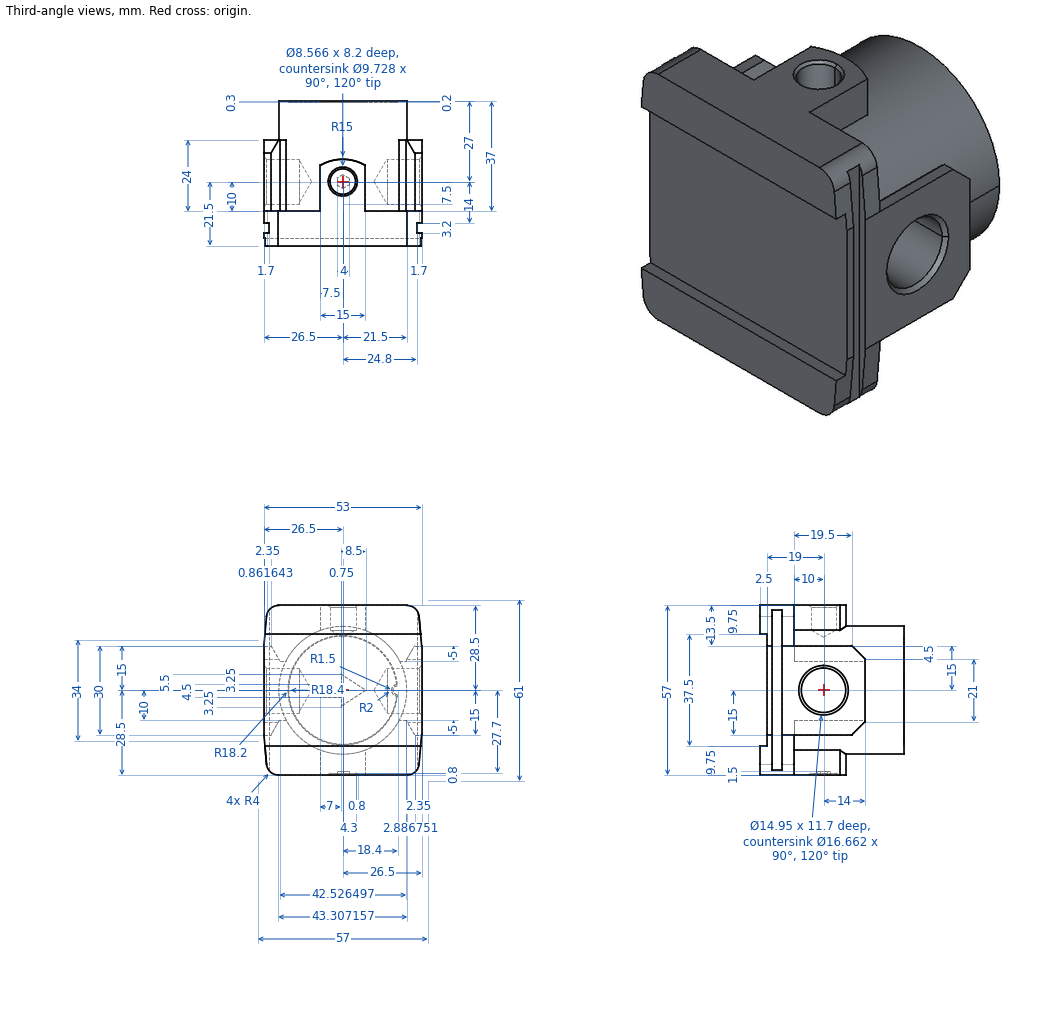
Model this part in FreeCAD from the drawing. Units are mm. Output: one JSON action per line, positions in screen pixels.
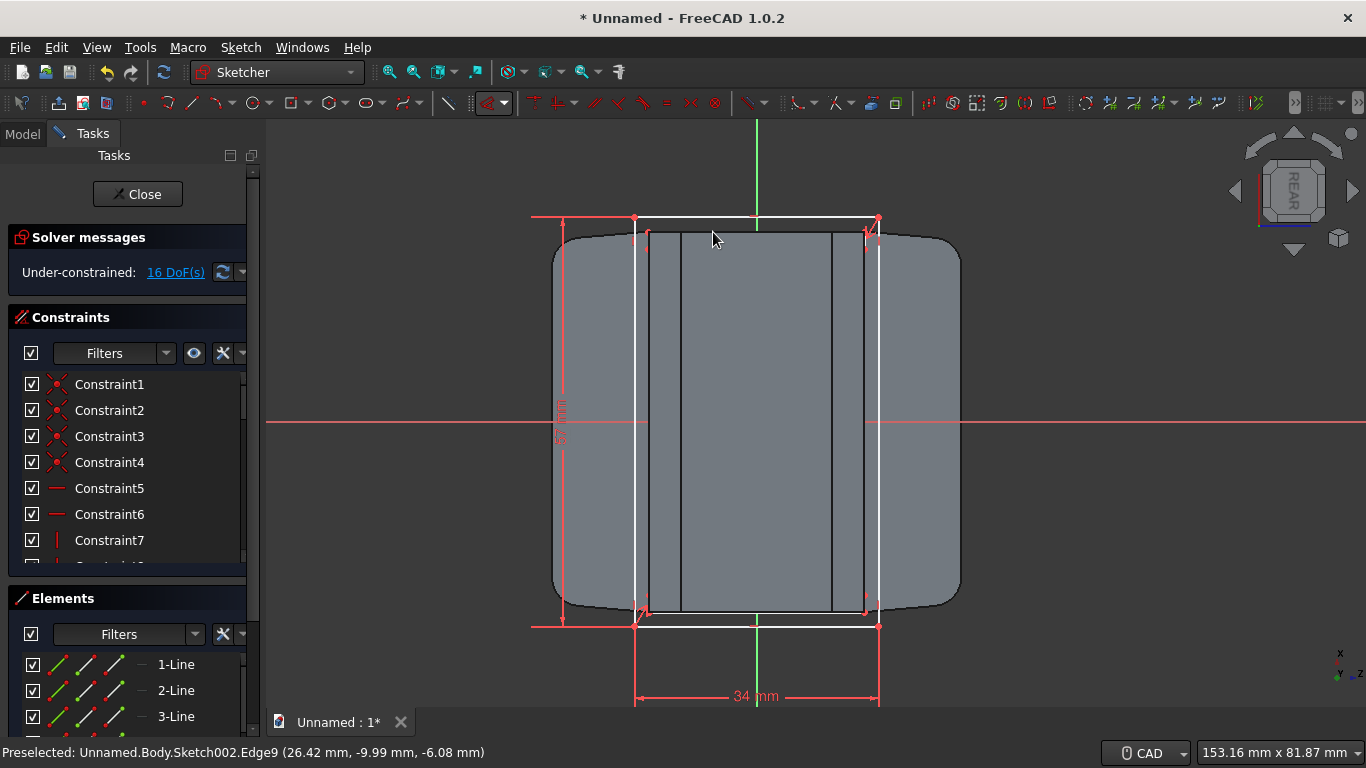
{"action": "left_click", "coordinate": [506, 104]}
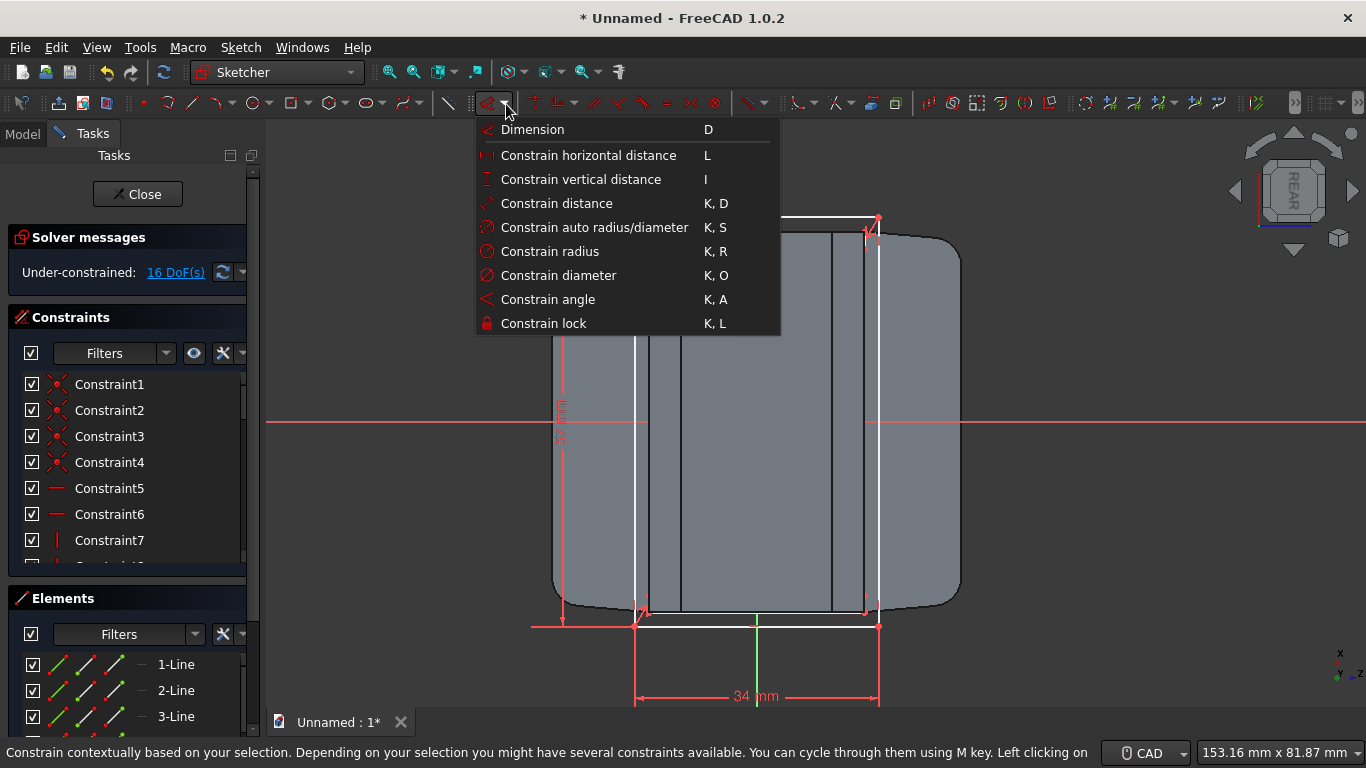
{"action": "left_click", "coordinate": [628, 155]}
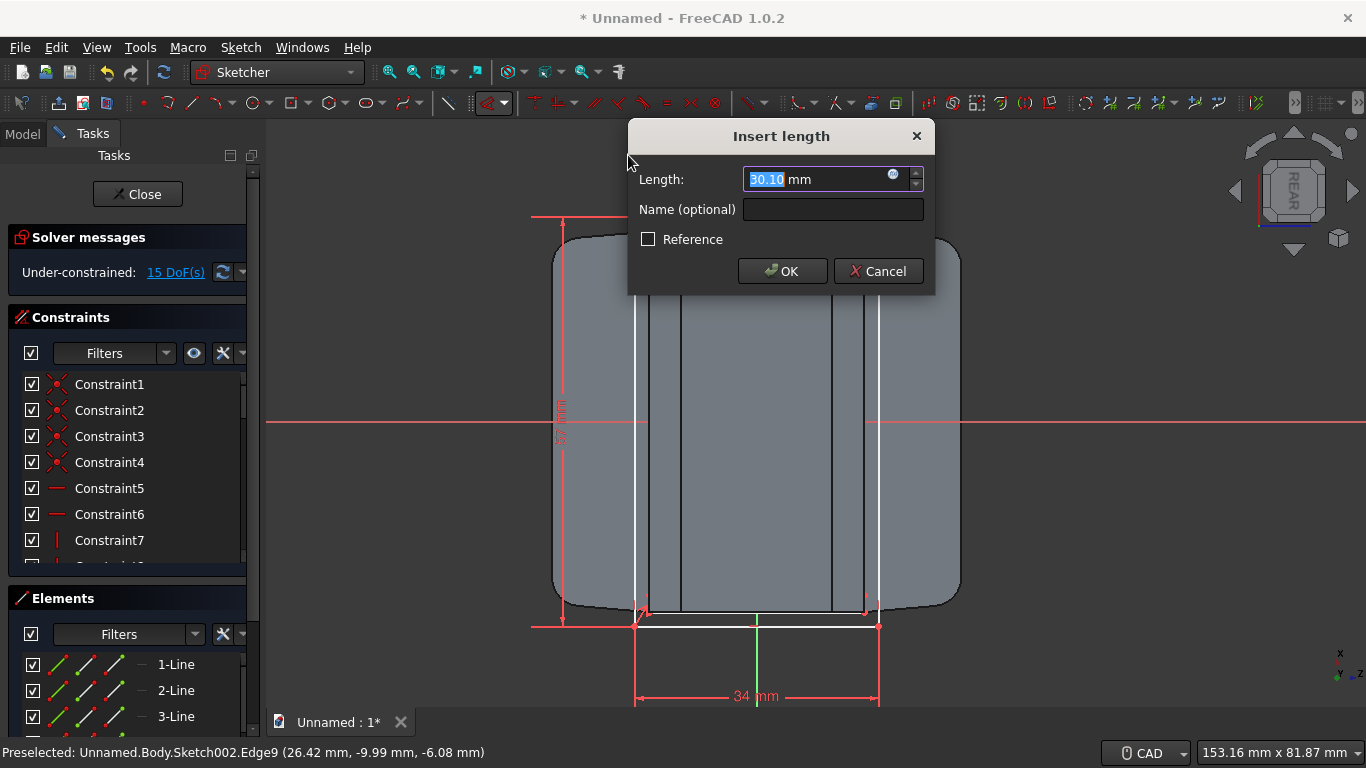
{"action": "type", "text": "30"}
{"action": "key", "text": "Return"}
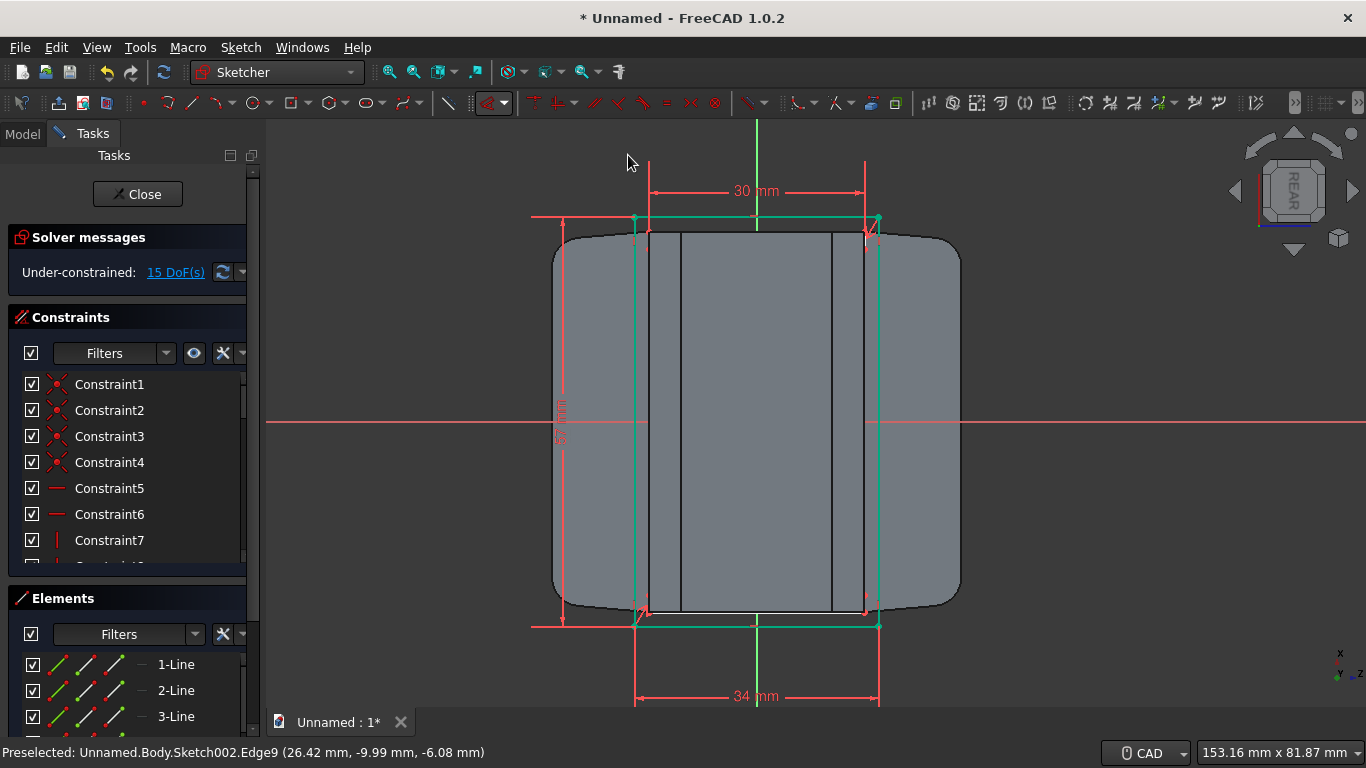
{"action": "left_click", "coordinate": [800, 613]}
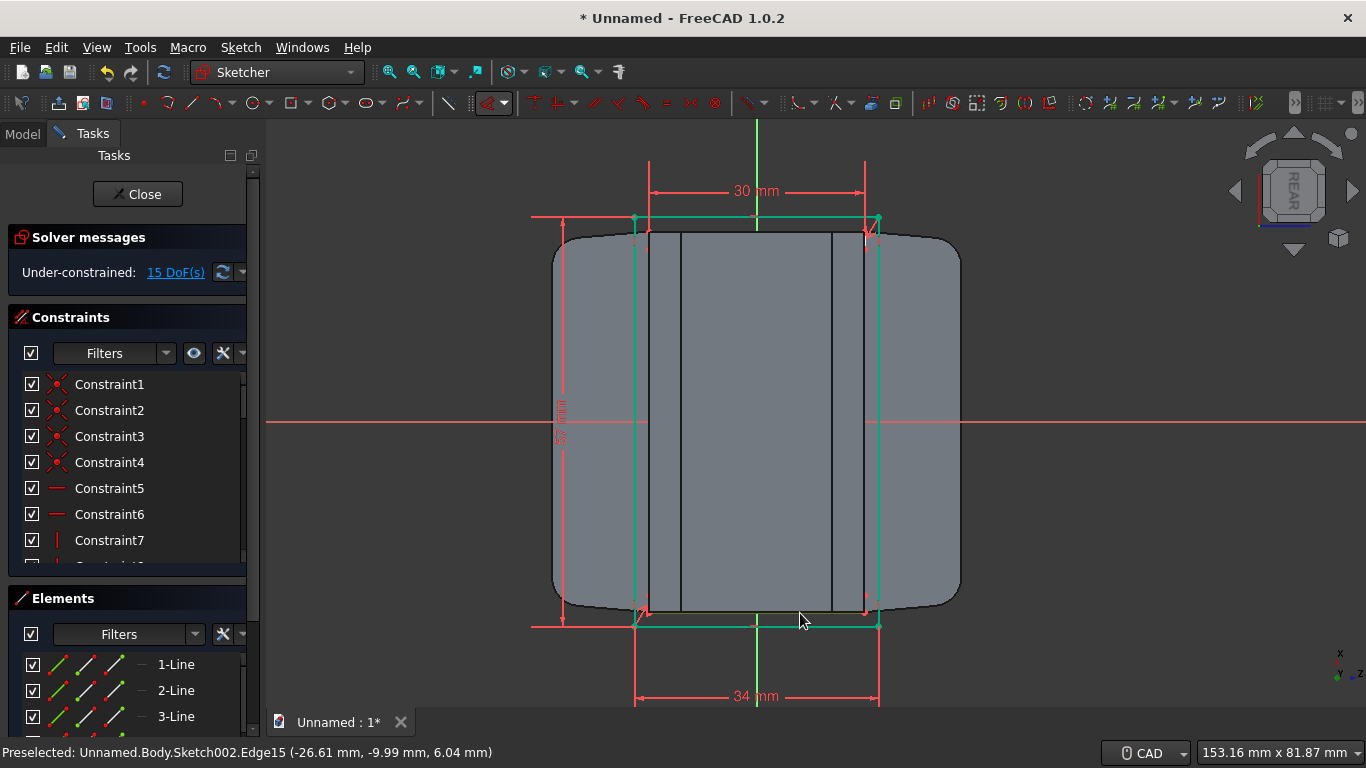
{"action": "left_click", "coordinate": [506, 104]}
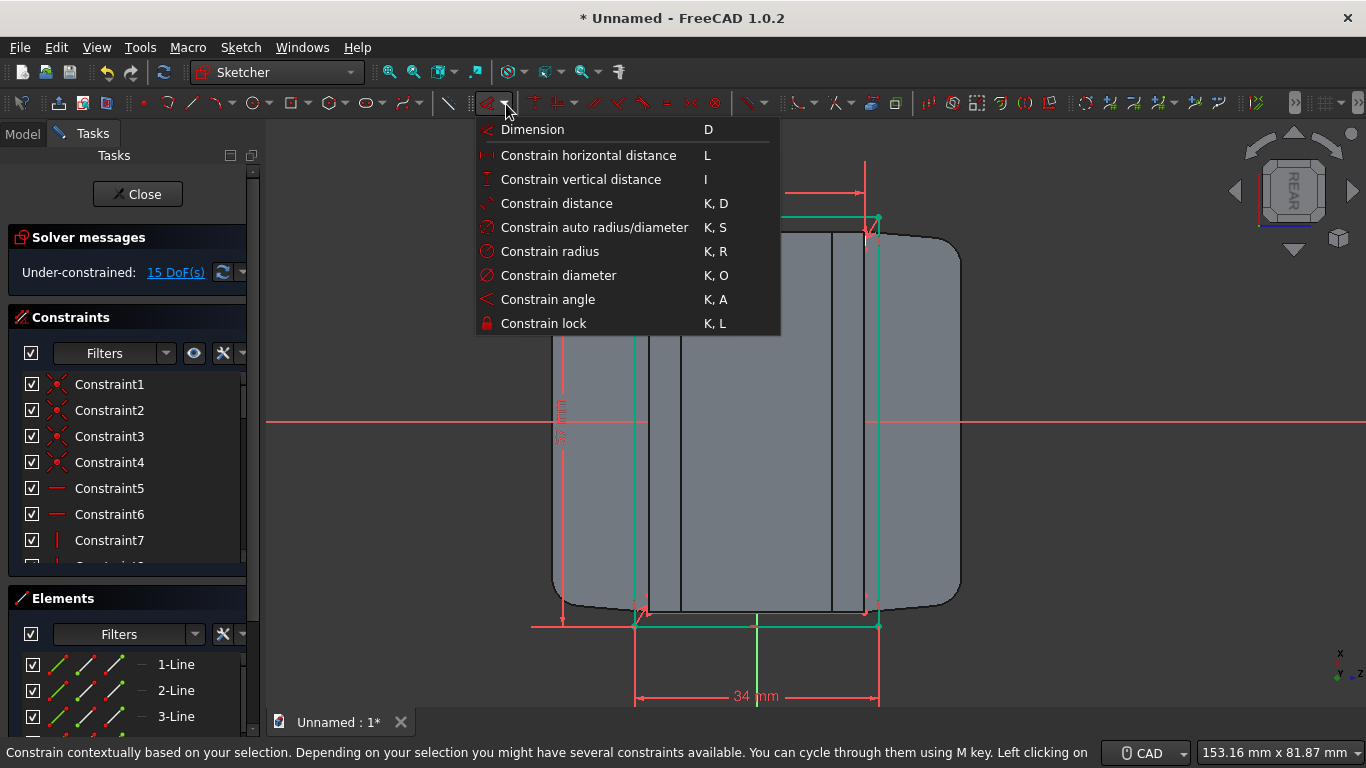
{"action": "left_click", "coordinate": [628, 155]}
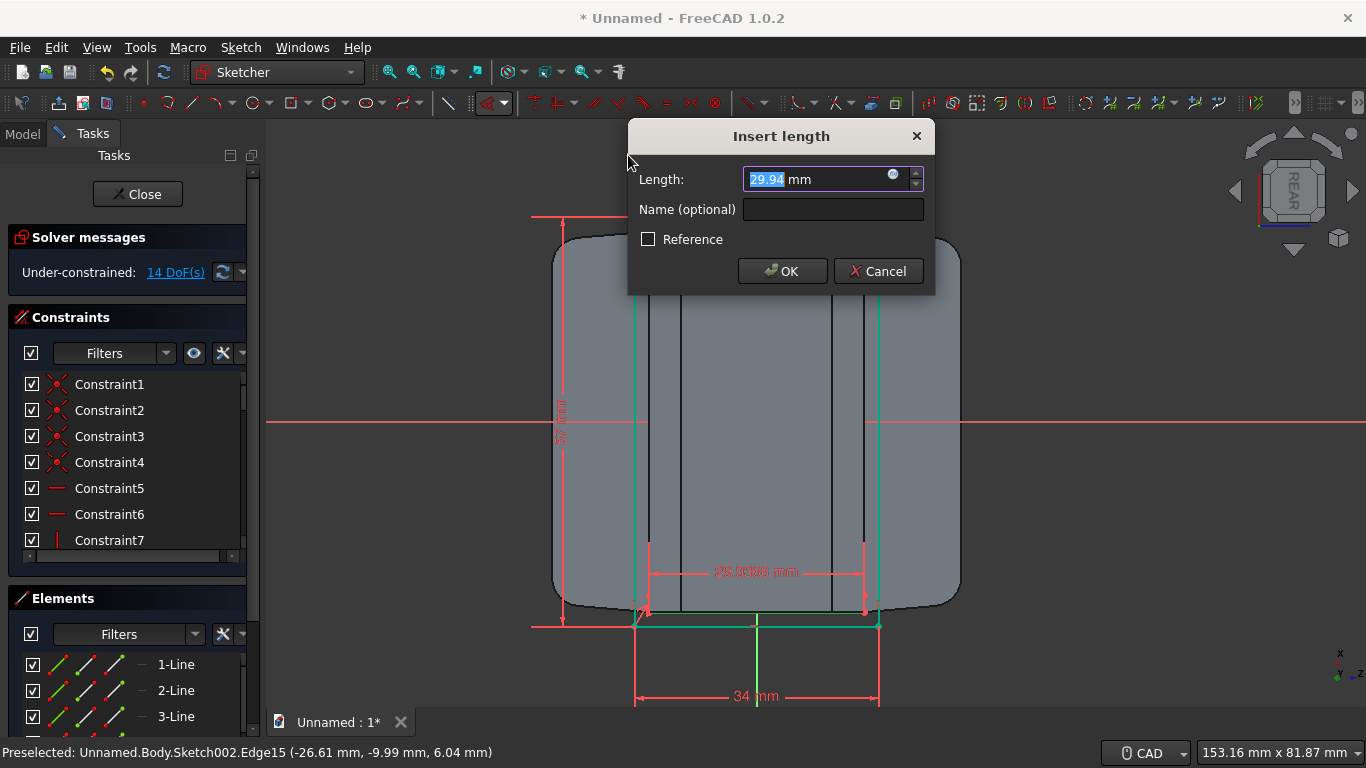
{"action": "type", "text": "30"}
{"action": "key", "text": "Return"}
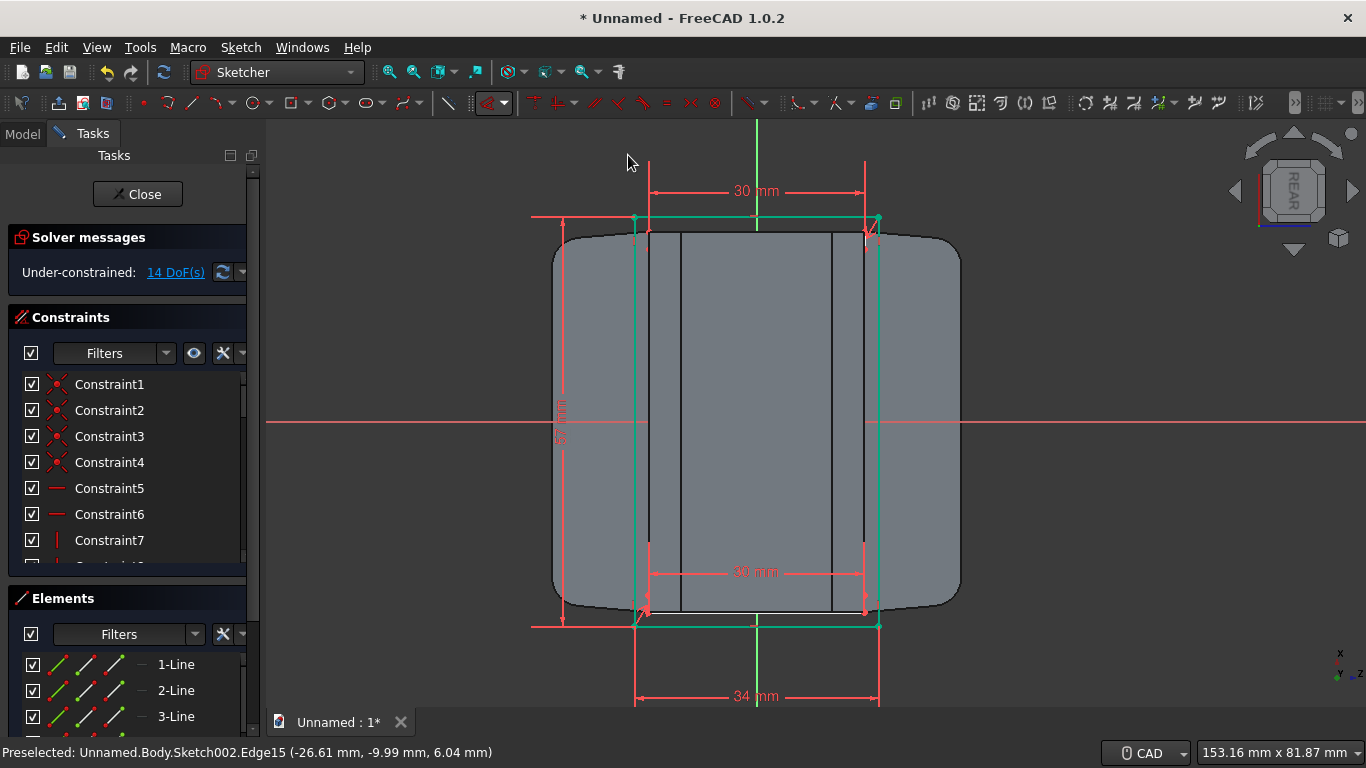
{"action": "left_click", "coordinate": [674, 264]}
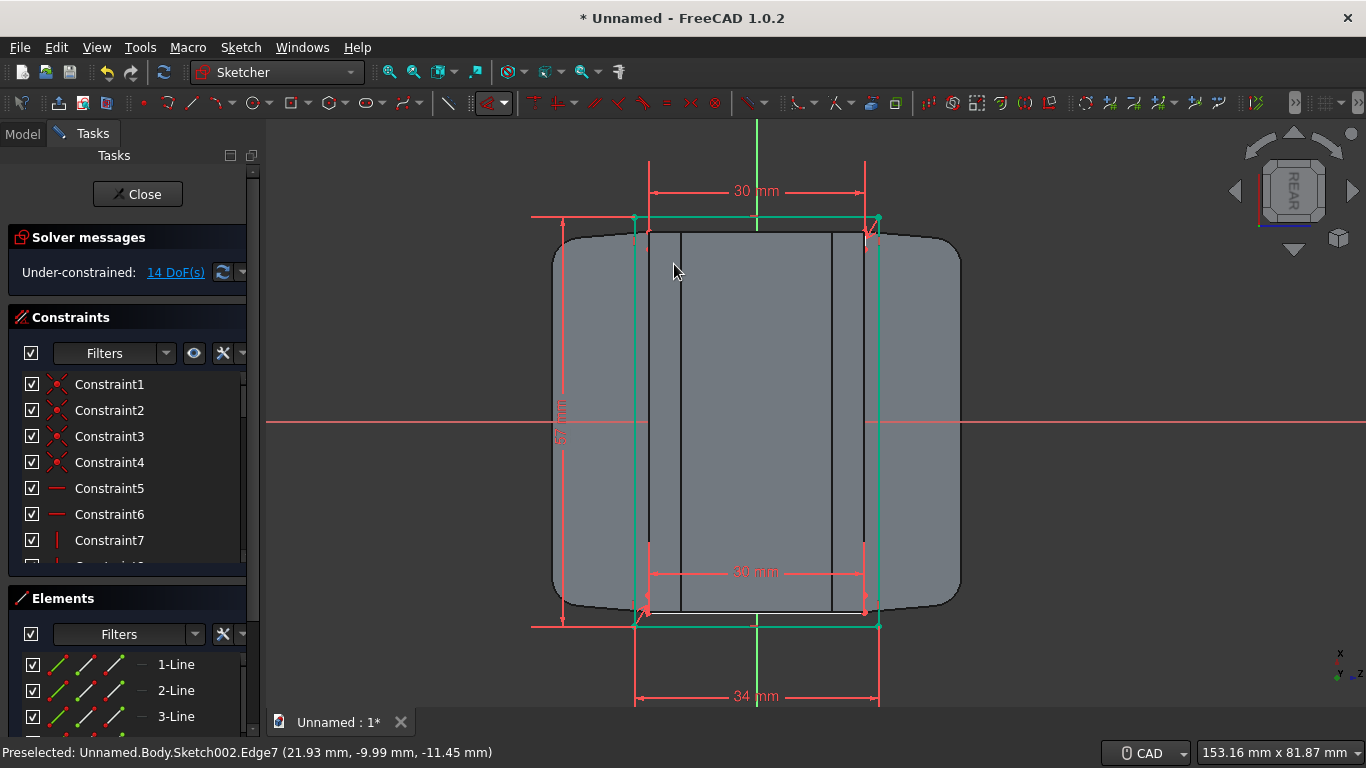
{"action": "left_click", "coordinate": [506, 104]}